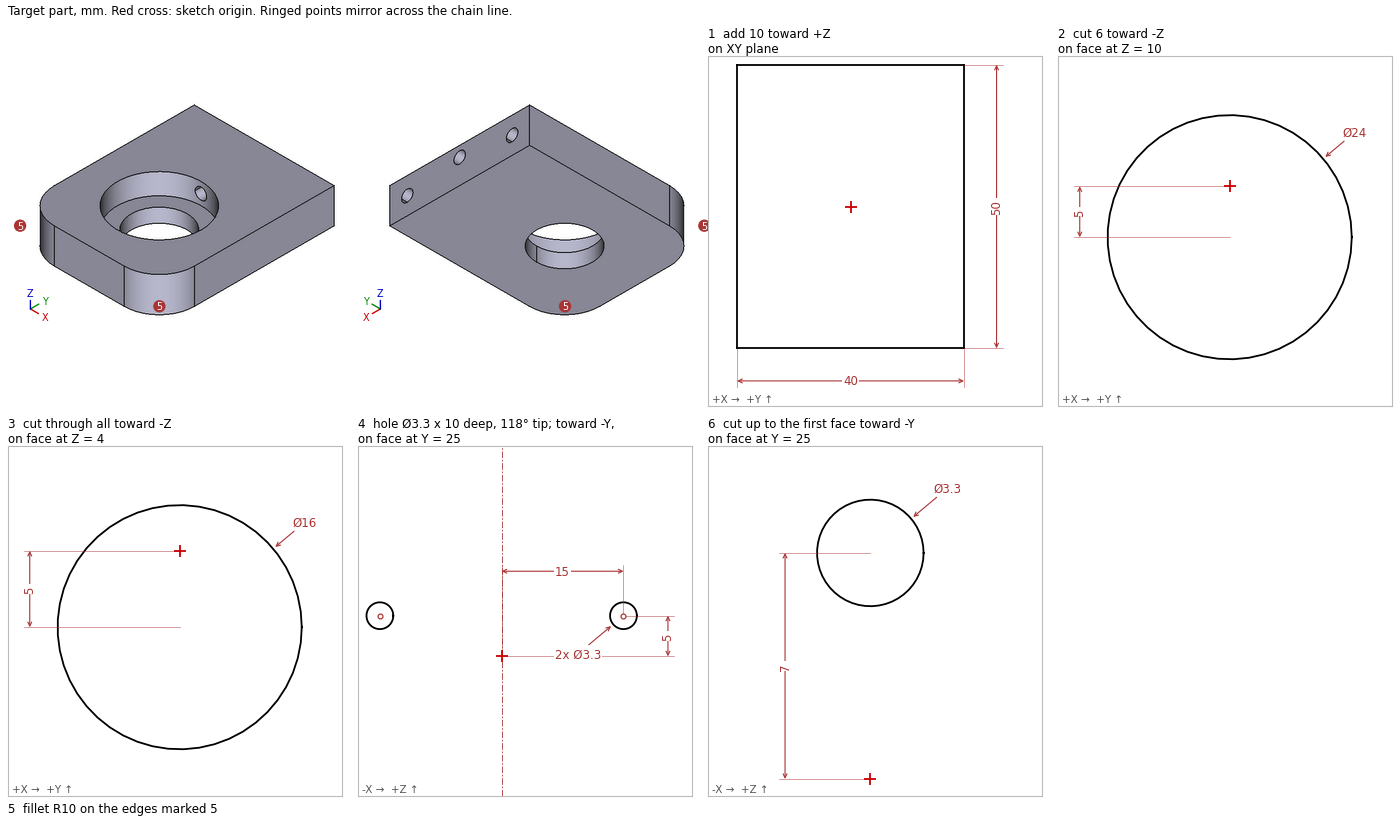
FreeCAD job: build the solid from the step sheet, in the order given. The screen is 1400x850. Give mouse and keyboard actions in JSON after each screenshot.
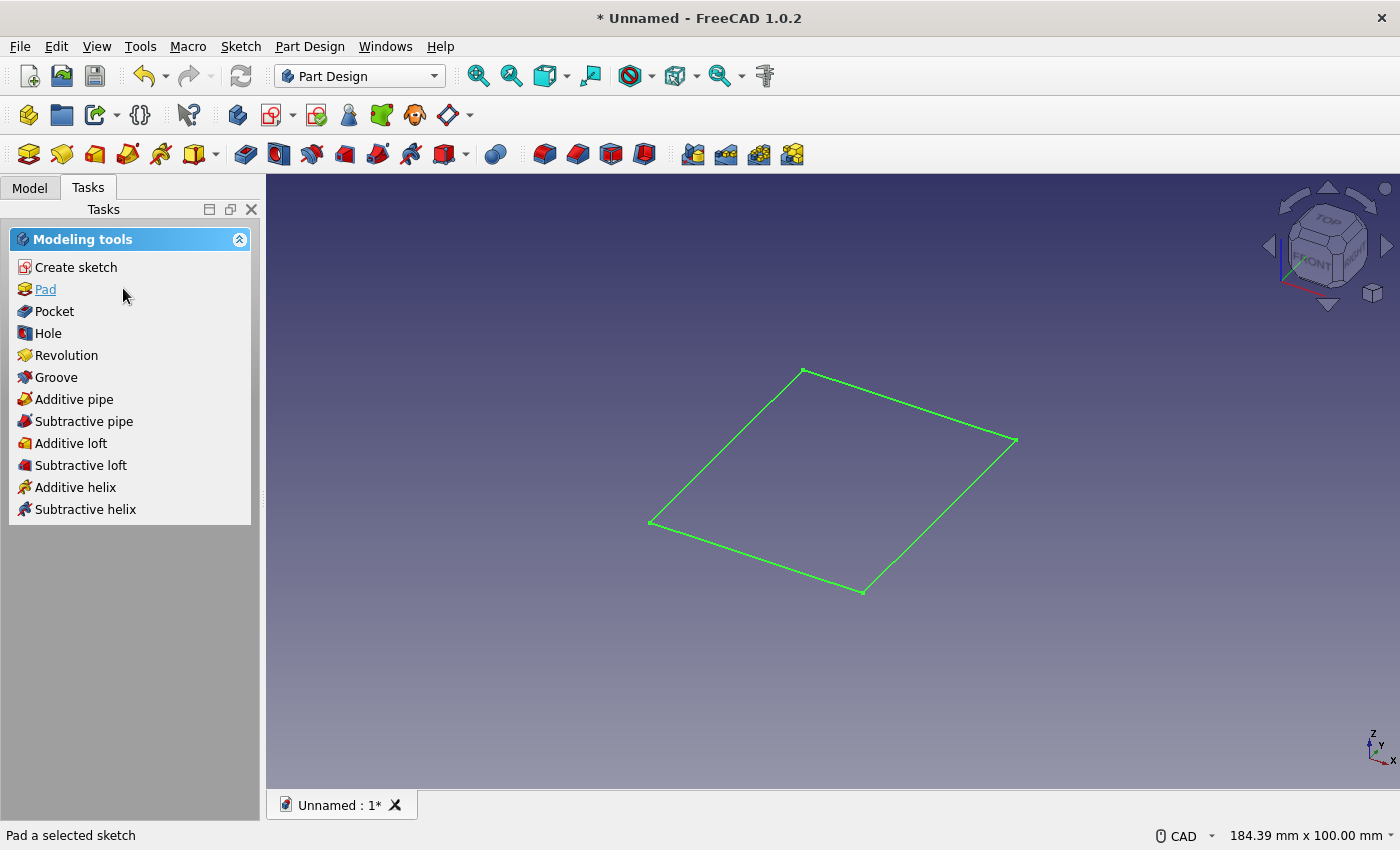
{"action": "left_click", "coordinate": [29, 154]}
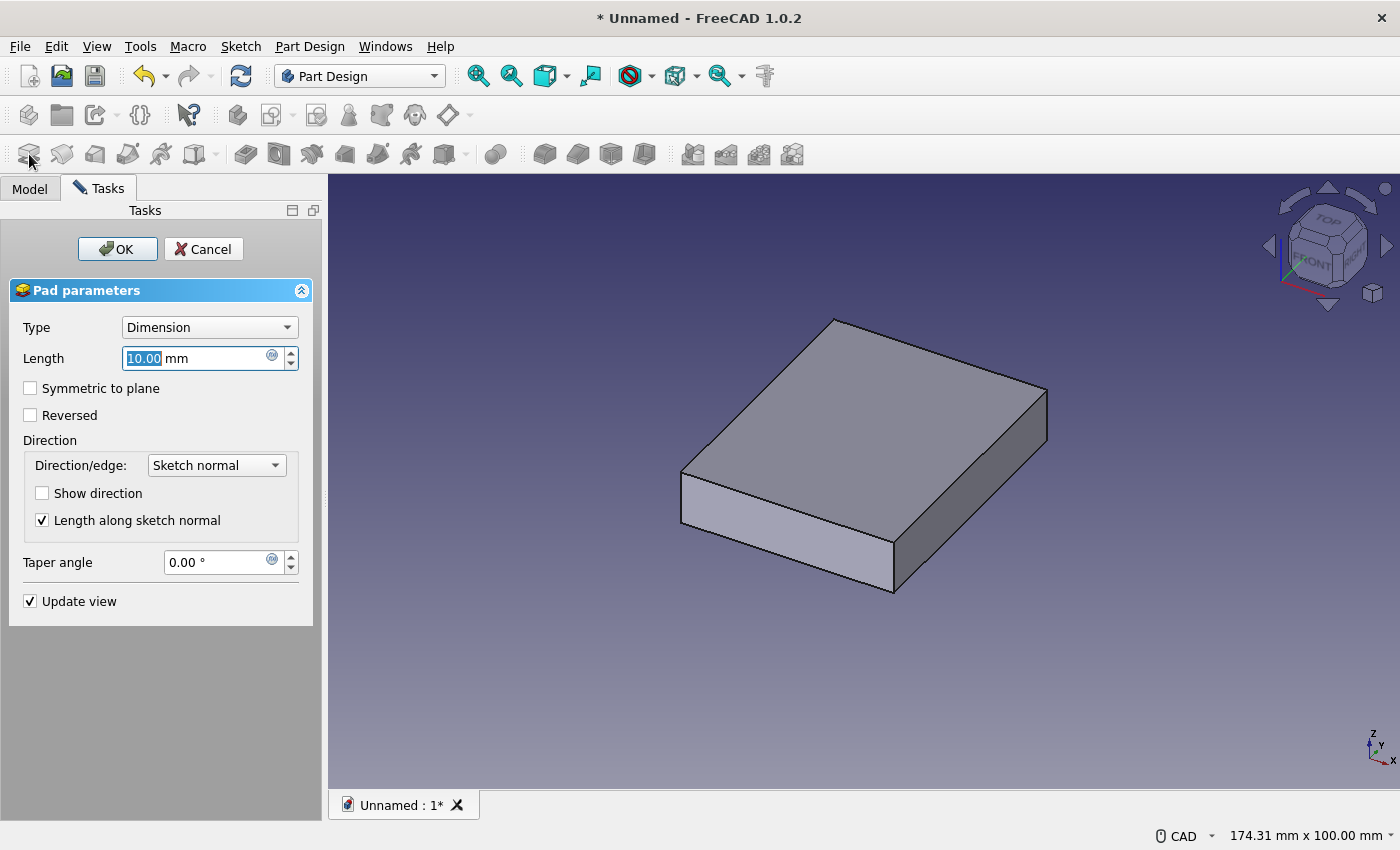
{"action": "type", "text": "10"}
{"action": "key", "text": "Tab"}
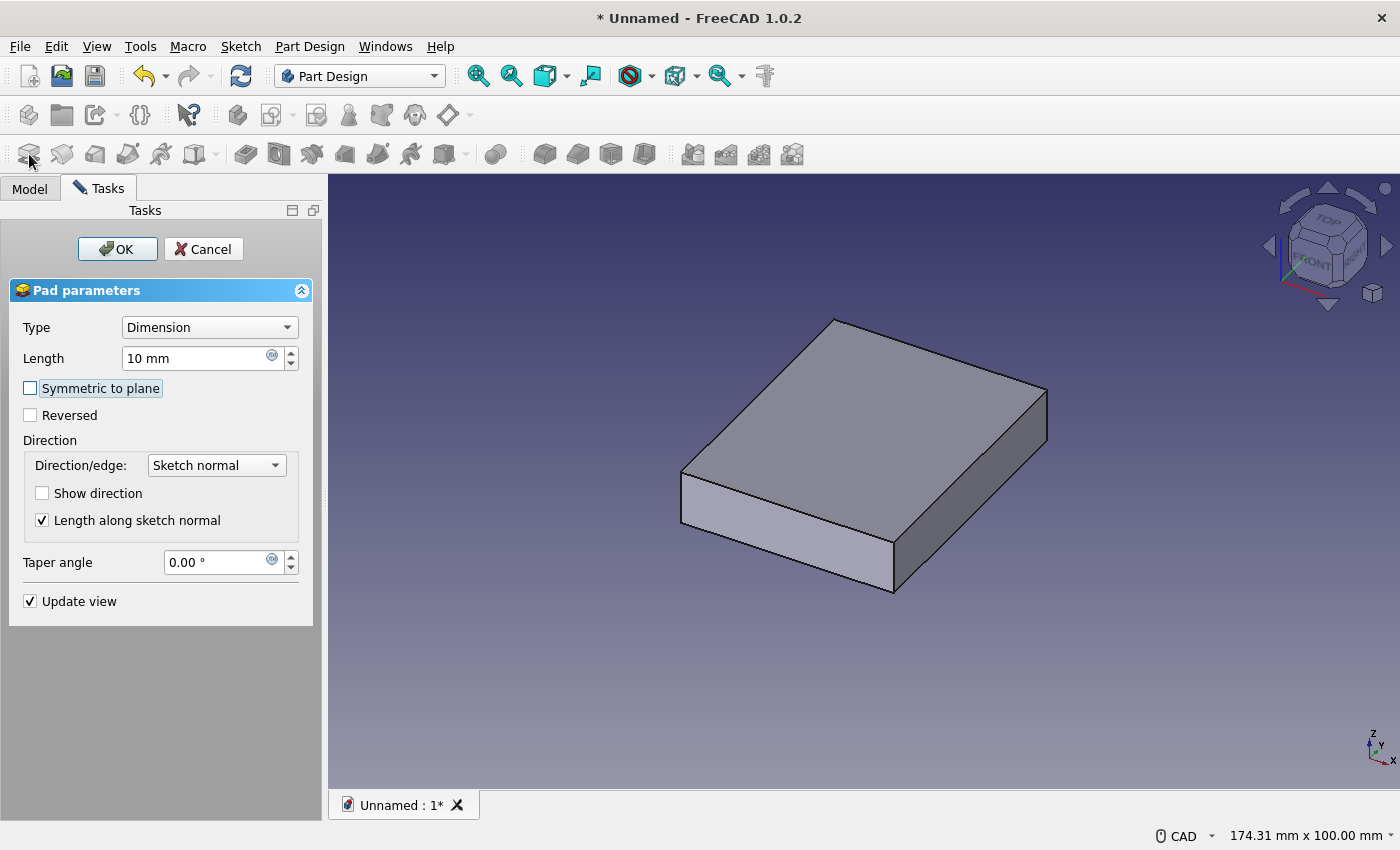
{"action": "left_click", "coordinate": [118, 249]}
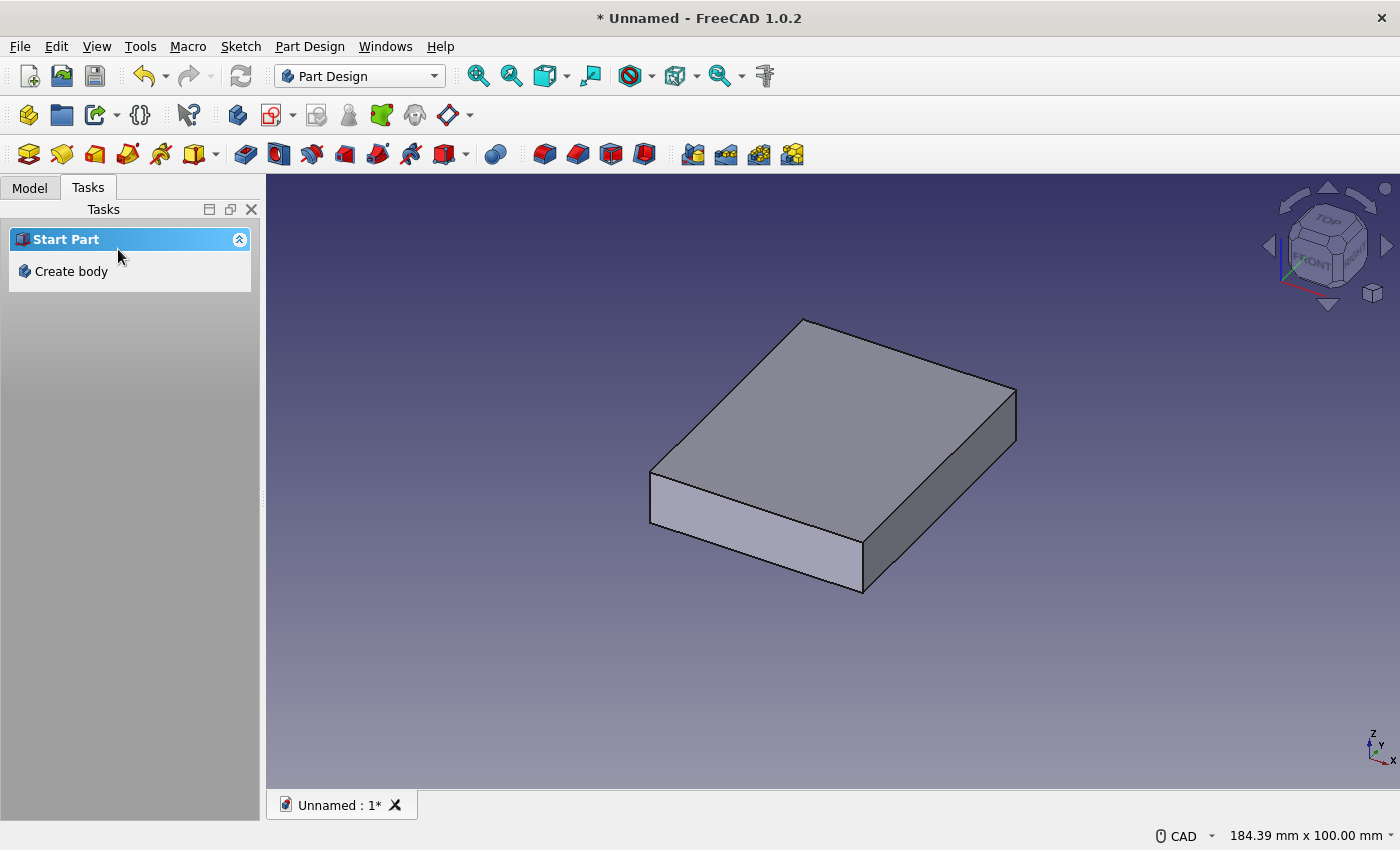
{"action": "left_click", "coordinate": [479, 76]}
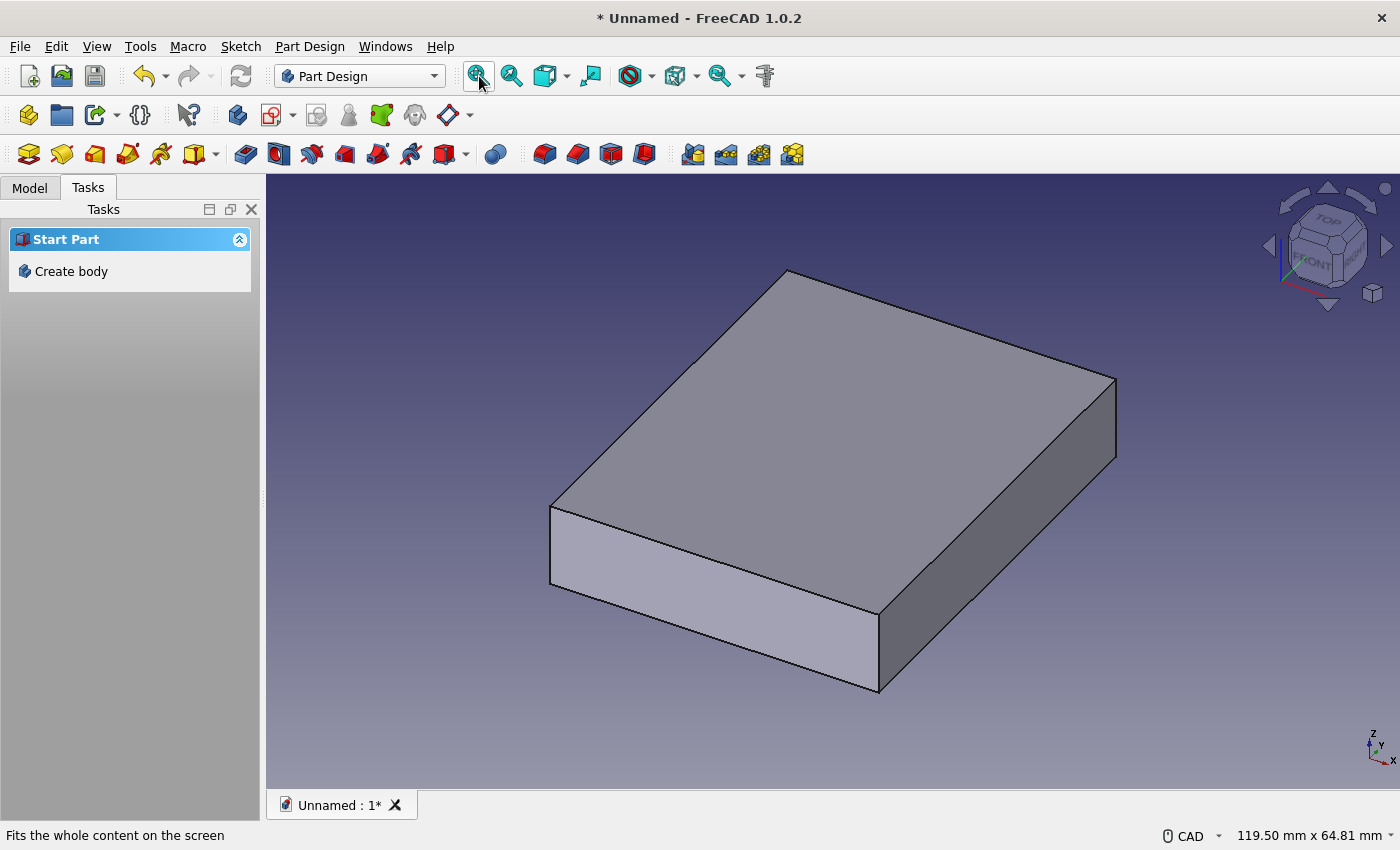
{"action": "left_click", "coordinate": [833, 442]}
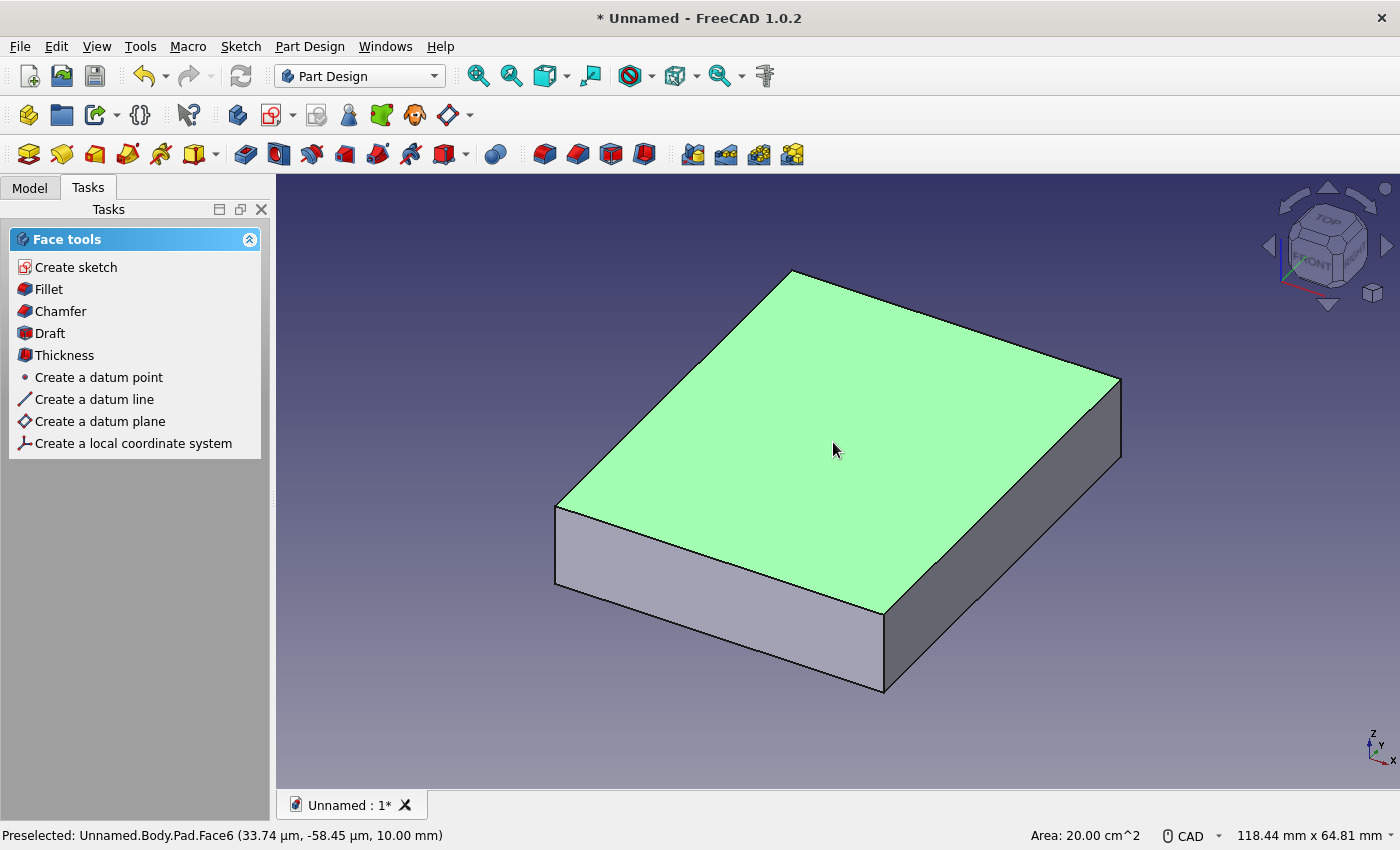
{"action": "left_click", "coordinate": [270, 116]}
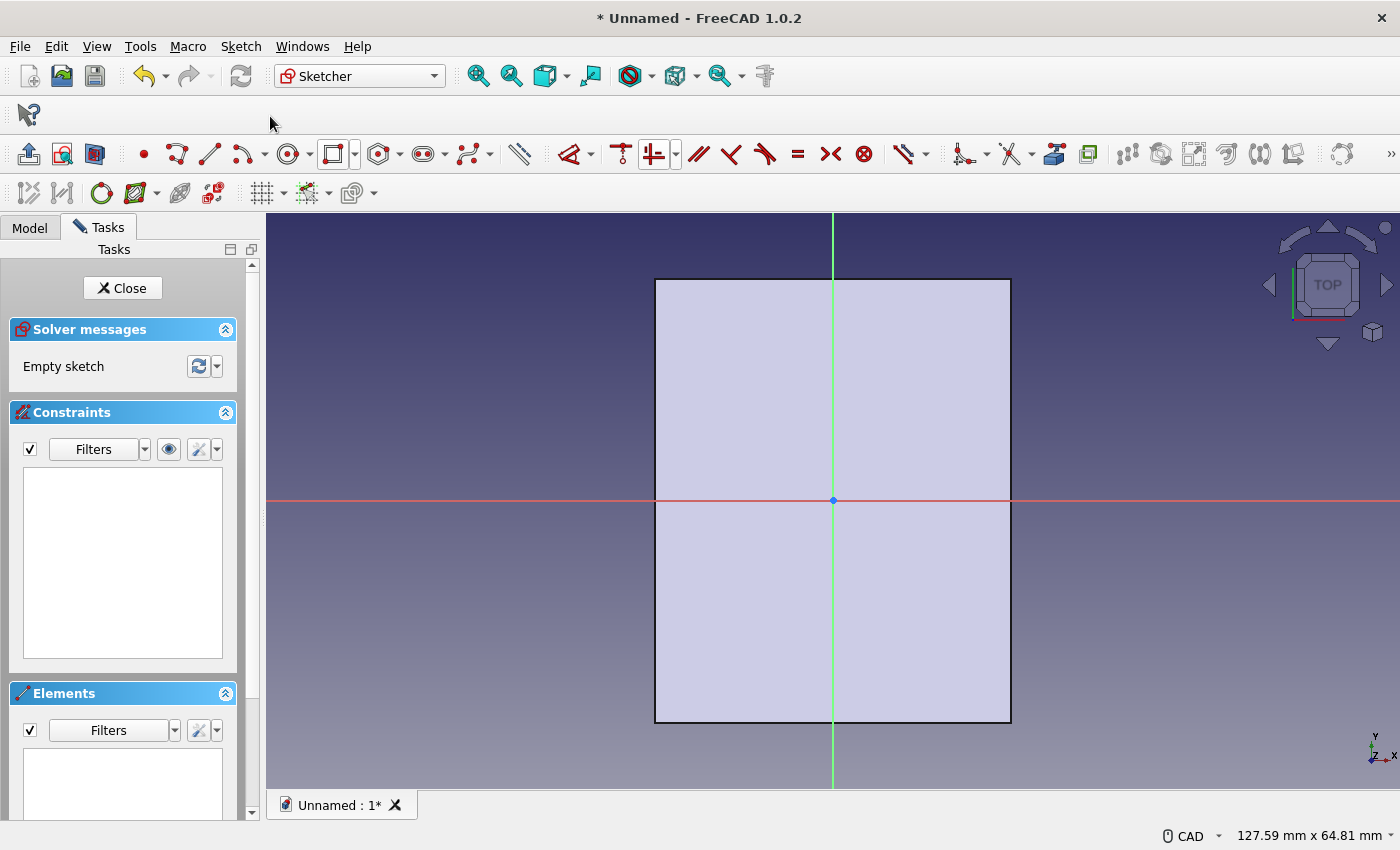
{"action": "scroll", "coordinate": [916, 599], "scroll_direction": "up", "scroll_amount": 3}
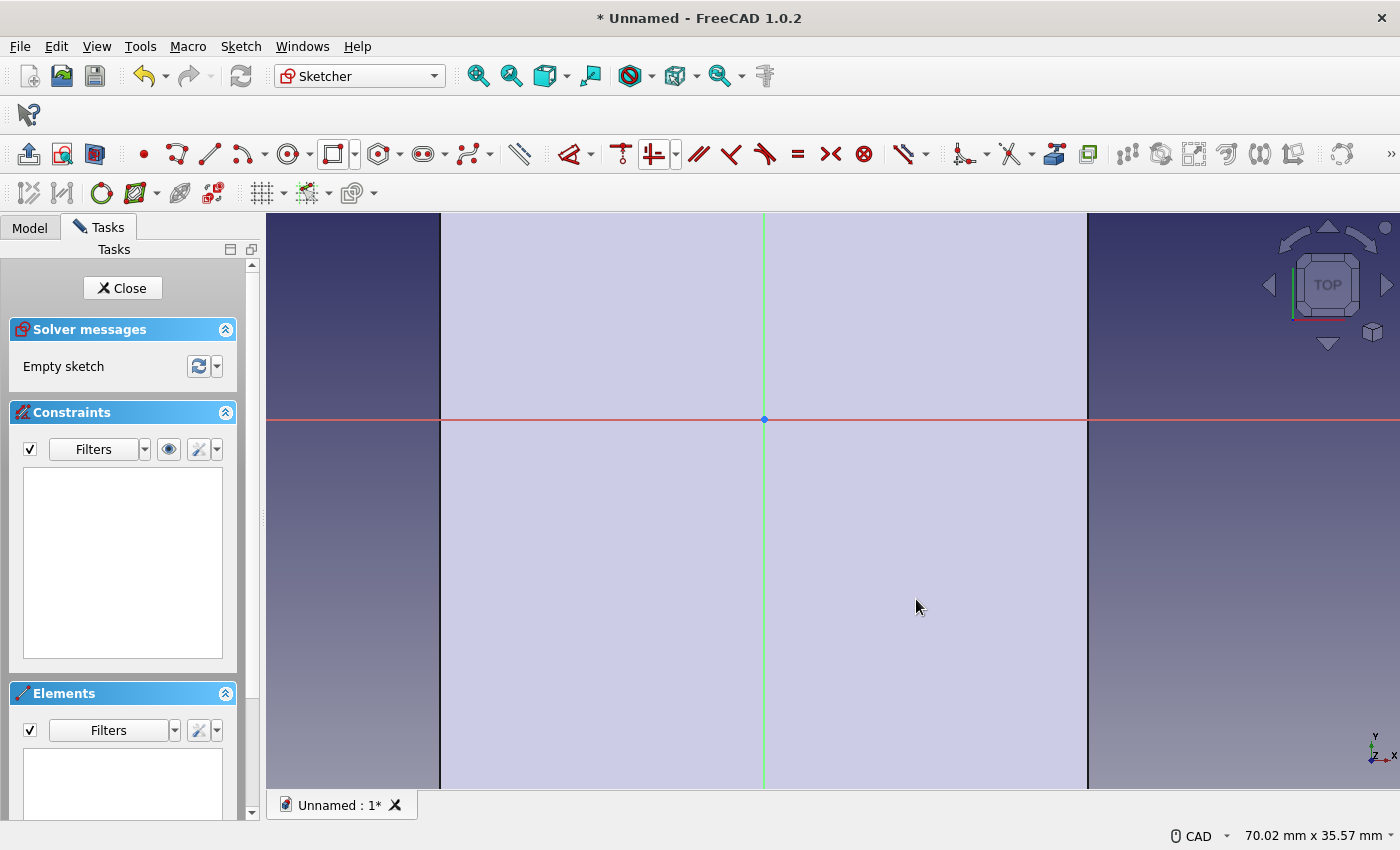
{"action": "left_click", "coordinate": [288, 154]}